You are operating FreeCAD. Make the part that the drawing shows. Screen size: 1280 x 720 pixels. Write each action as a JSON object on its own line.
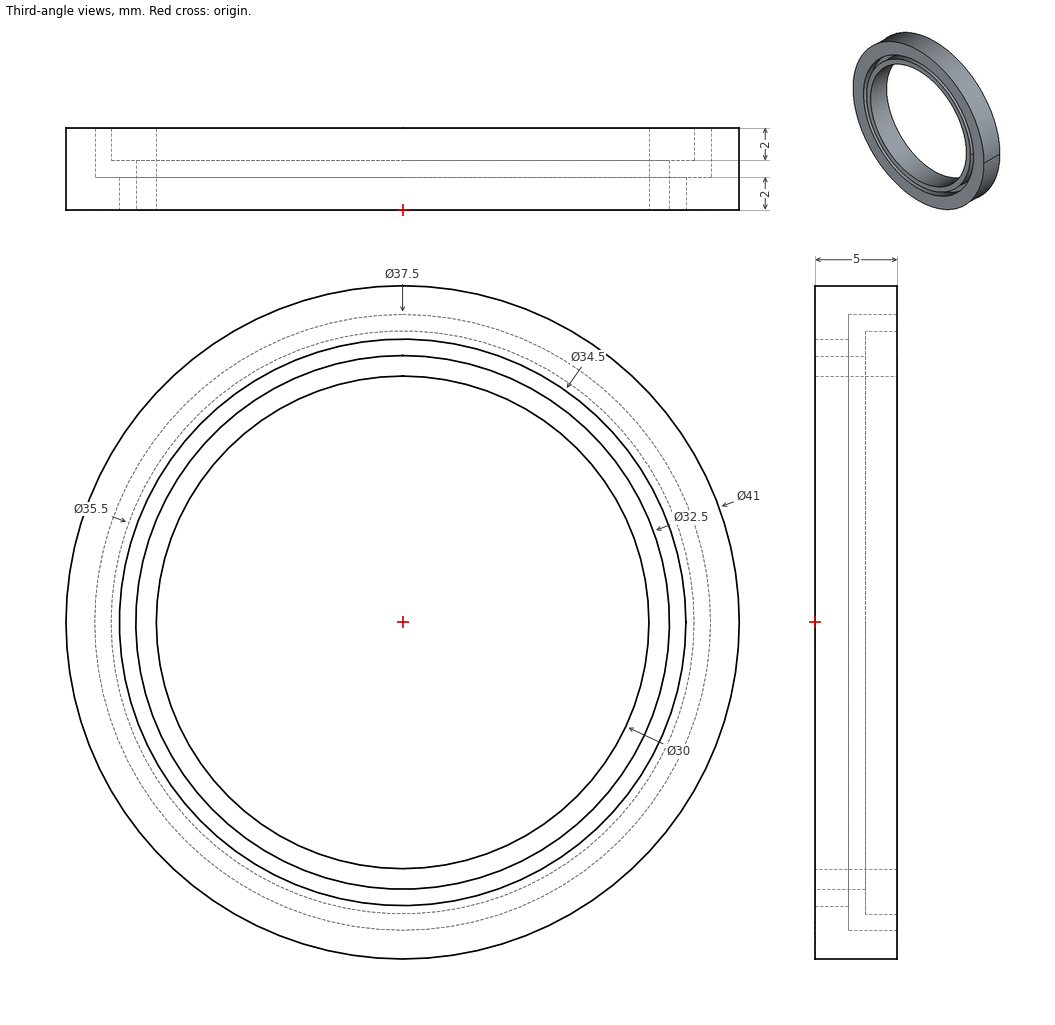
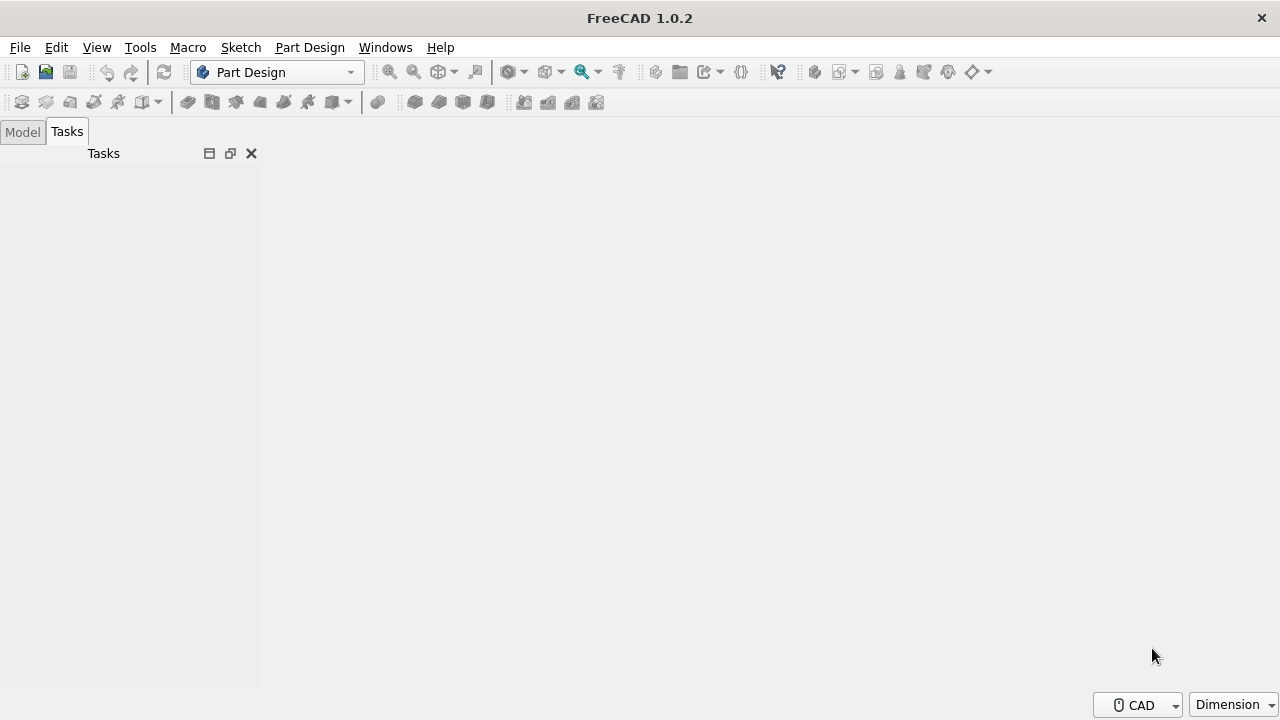
{"action": "key", "text": "ctrl+n"}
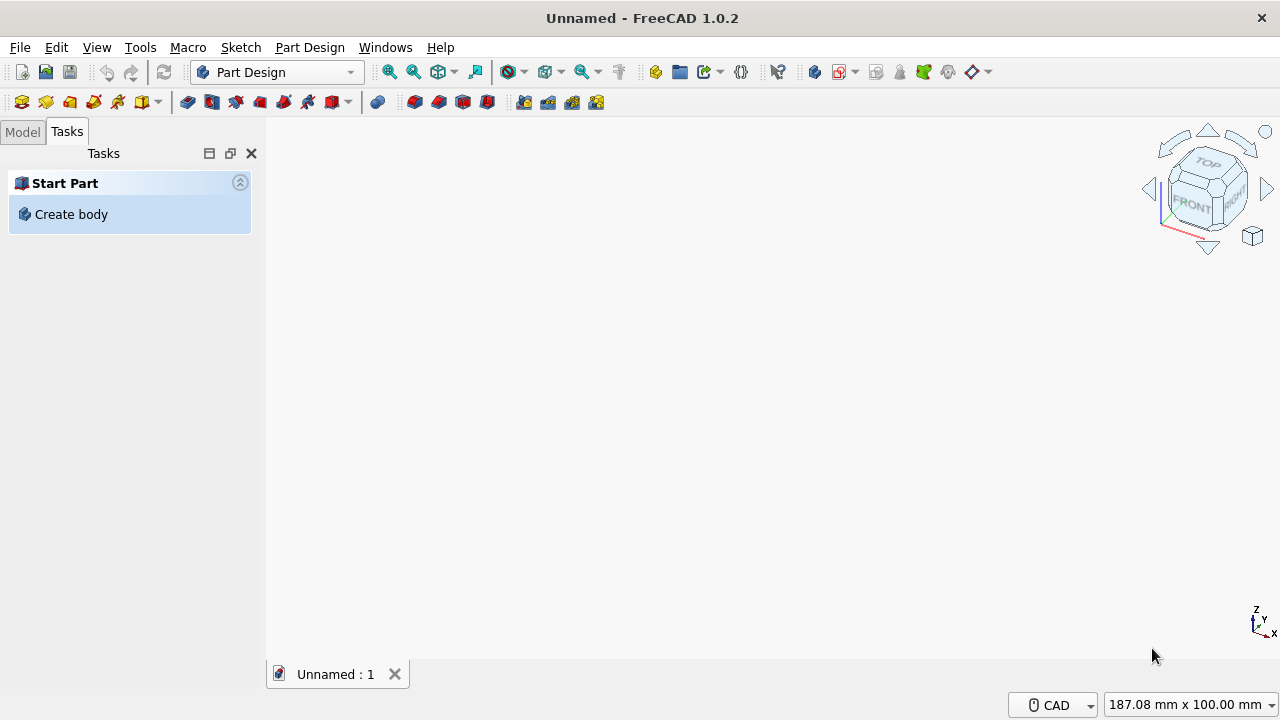
{"action": "left_click", "coordinate": [840, 72]}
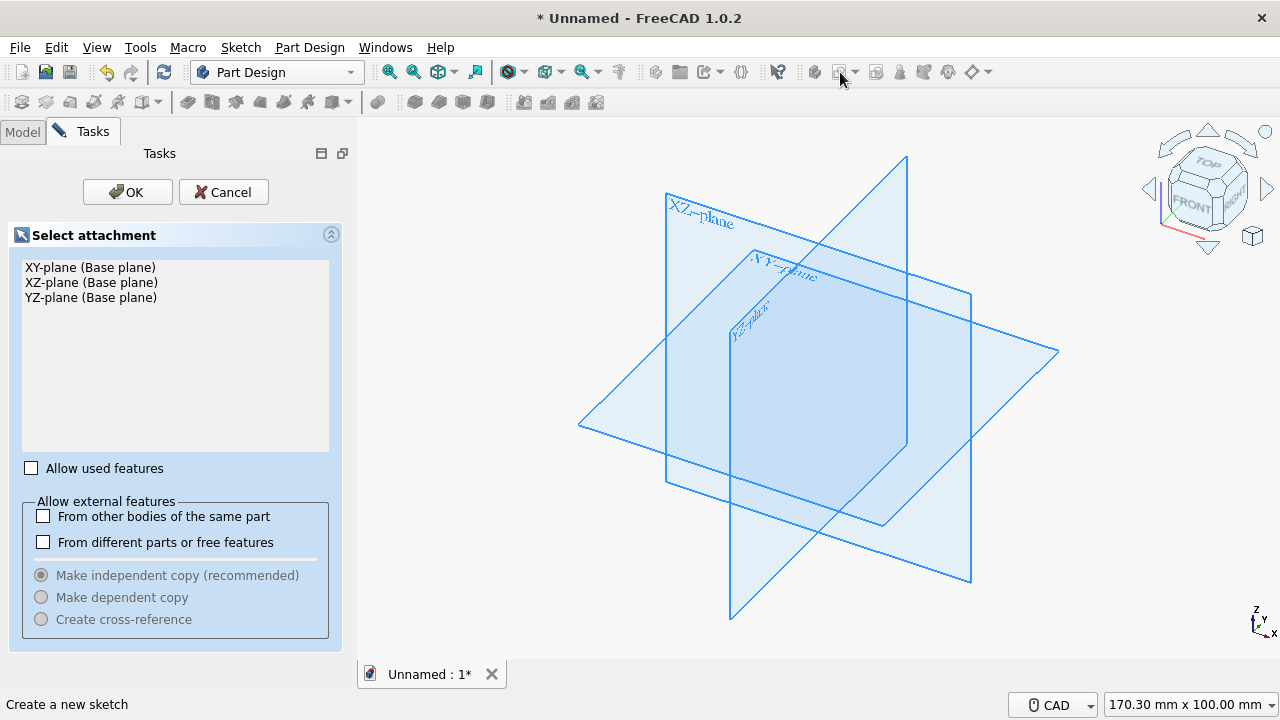
{"action": "left_click", "coordinate": [82, 282]}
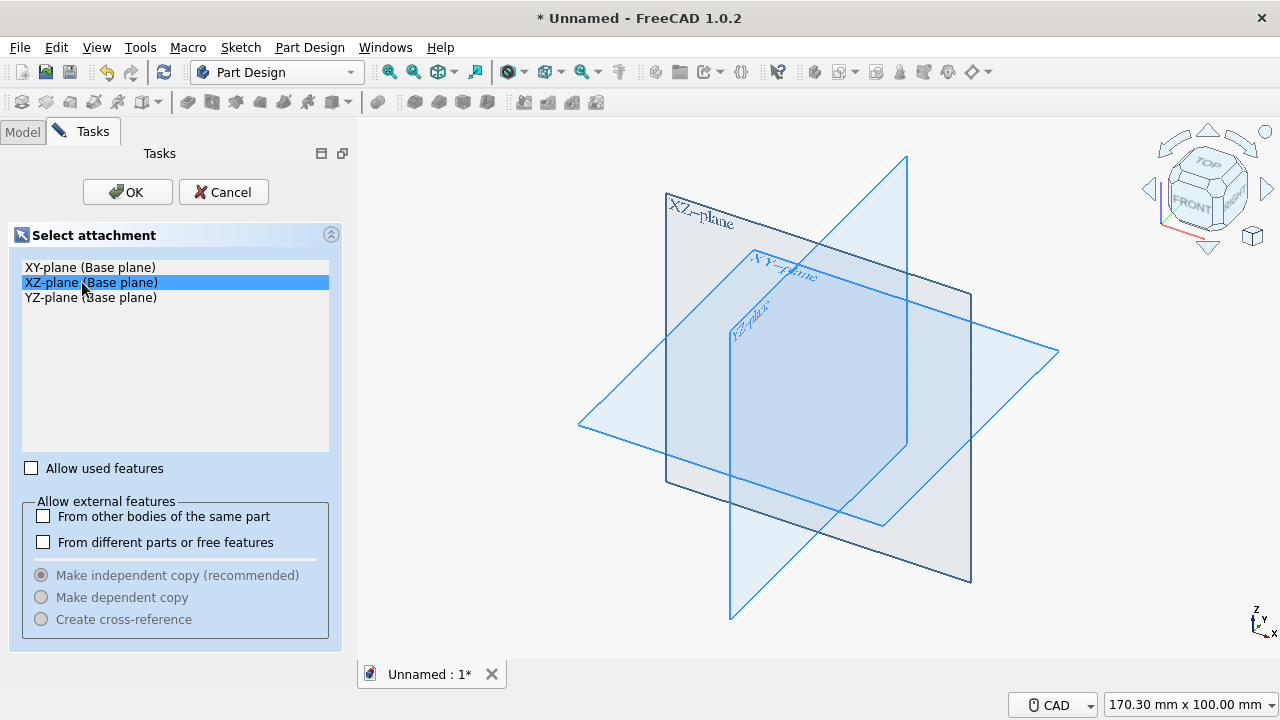
{"action": "left_click", "coordinate": [128, 192]}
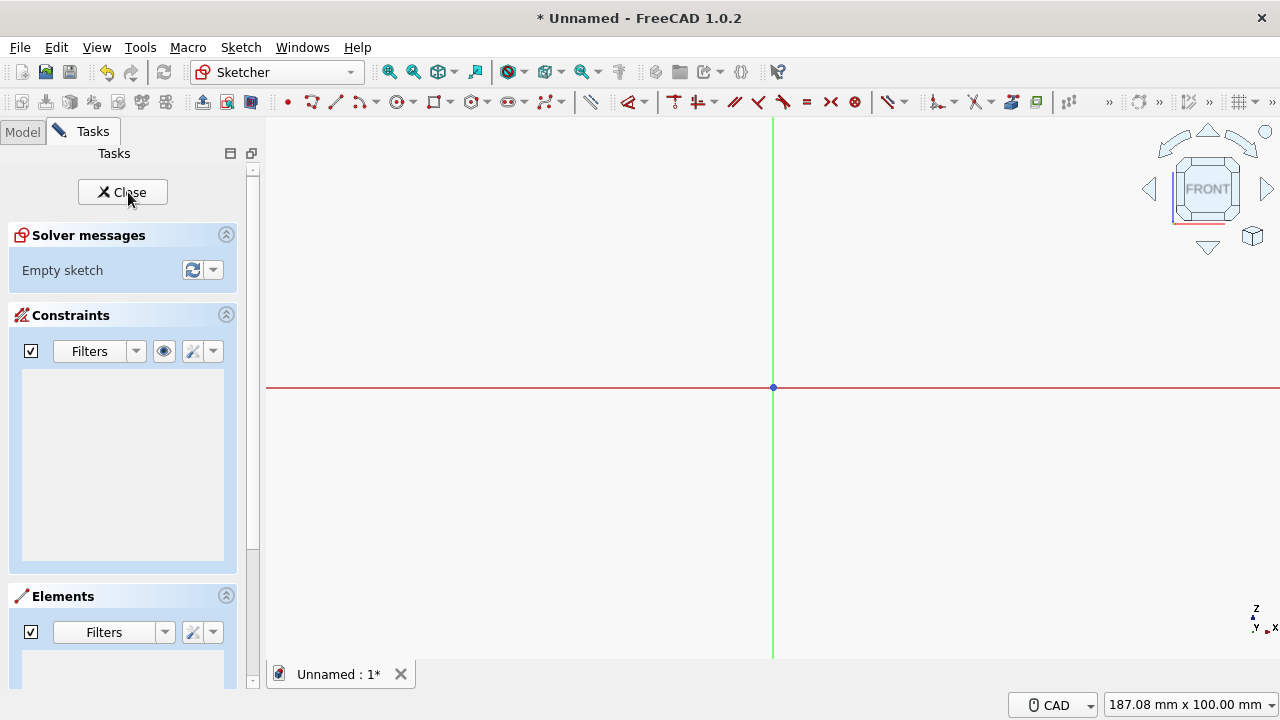
{"action": "scroll", "coordinate": [856, 388], "scroll_direction": "up", "scroll_amount": 3}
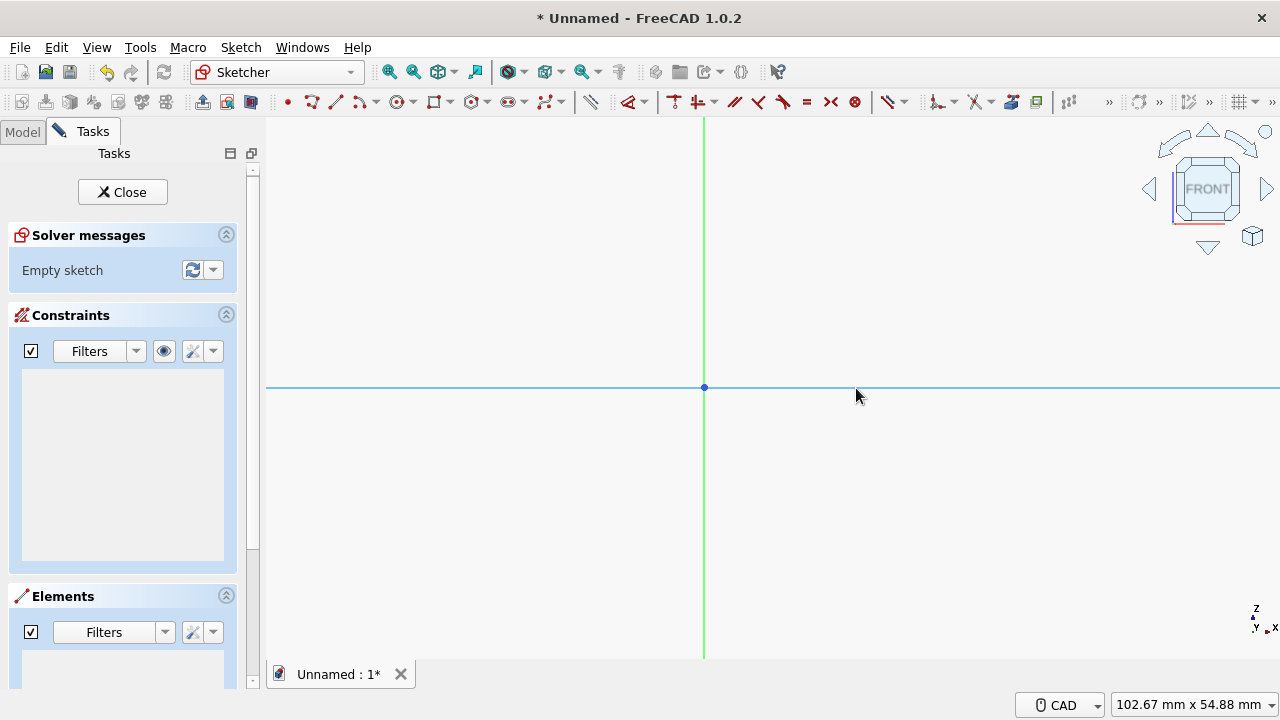
{"action": "key", "text": "g c"}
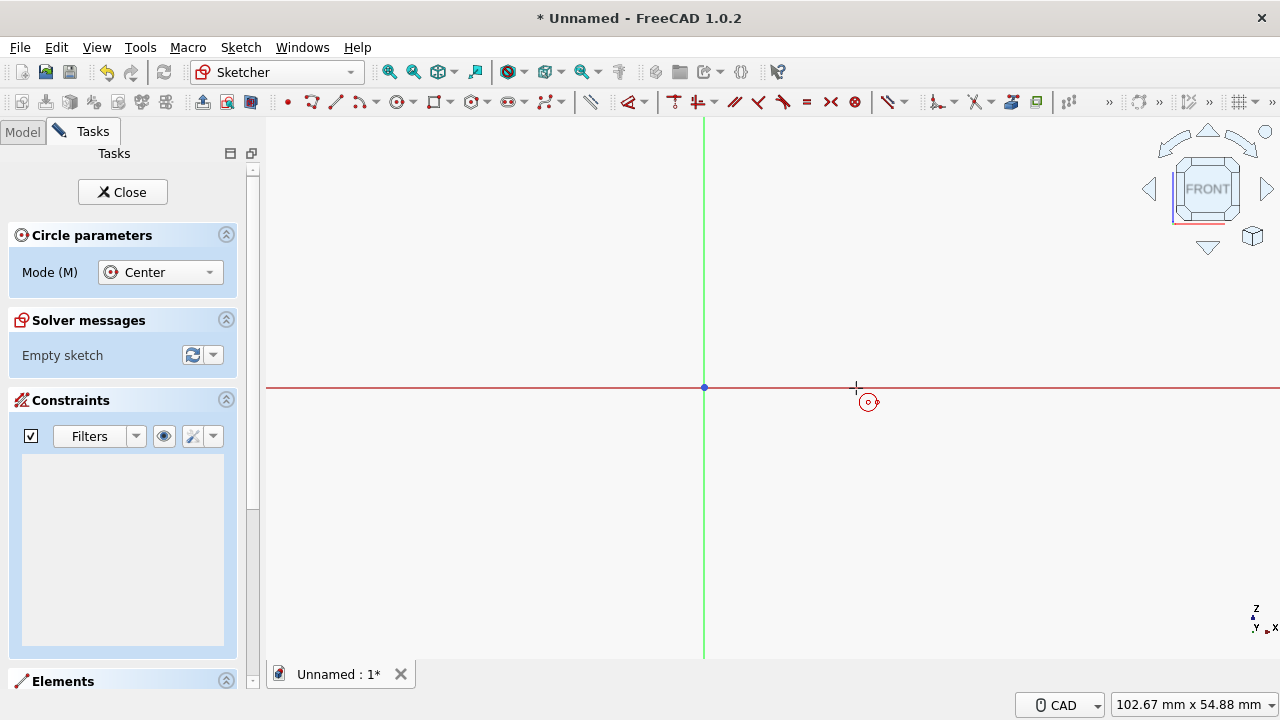
{"action": "left_click", "coordinate": [704, 388]}
{"action": "mouse_move", "coordinate": [818, 274]}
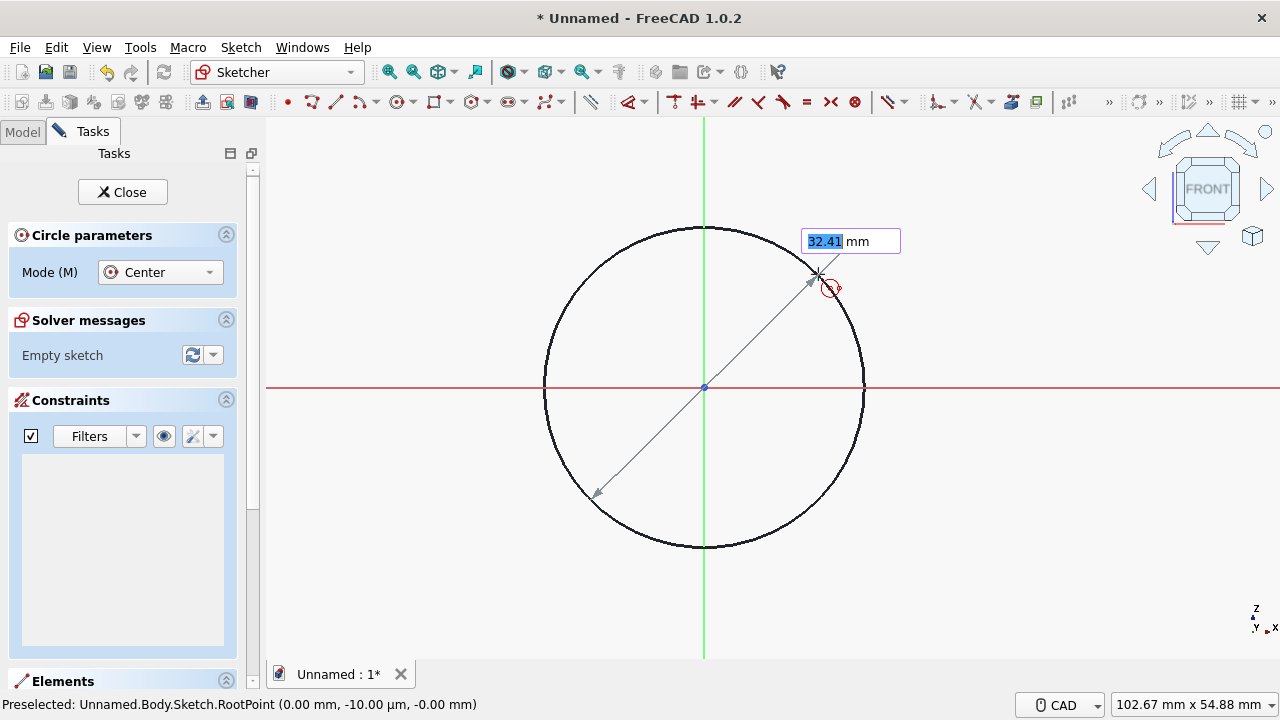
{"action": "type", "text": "32.5"}
{"action": "key", "text": "Return"}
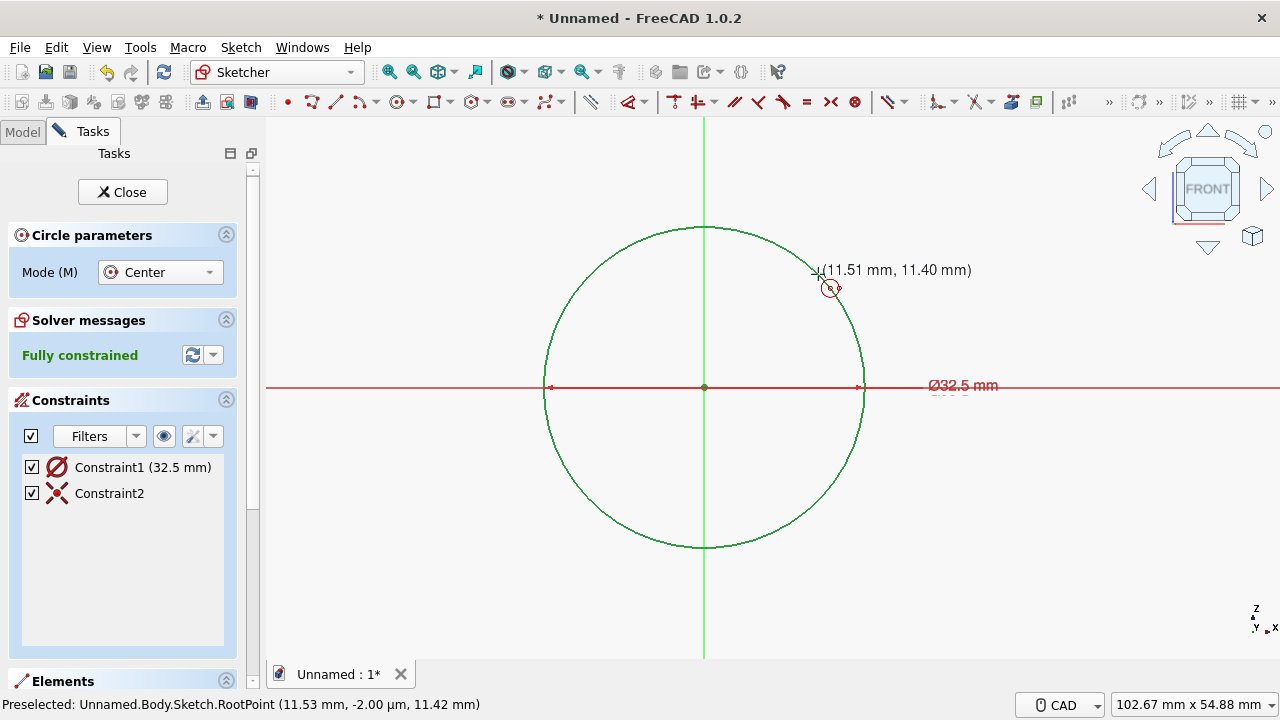
{"action": "left_click", "coordinate": [704, 388]}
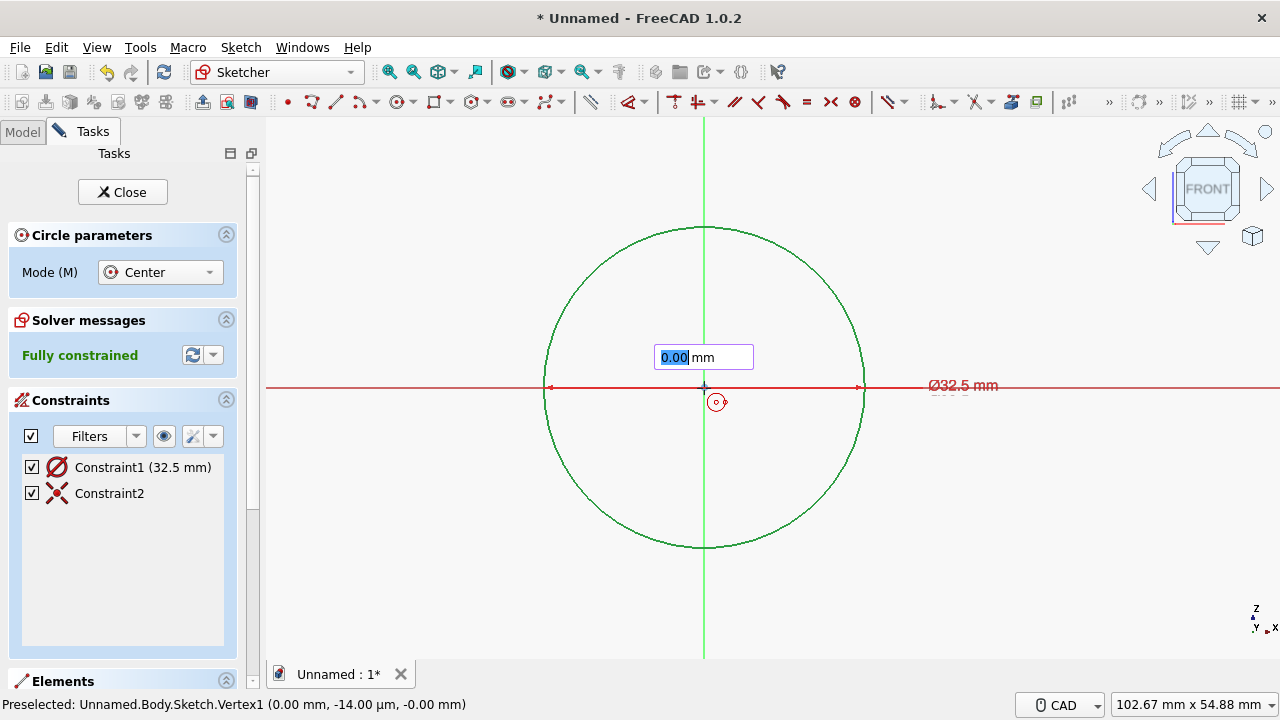
{"action": "scroll", "coordinate": [809, 283], "scroll_direction": "up", "scroll_amount": 2}
{"action": "mouse_move", "coordinate": [809, 283]}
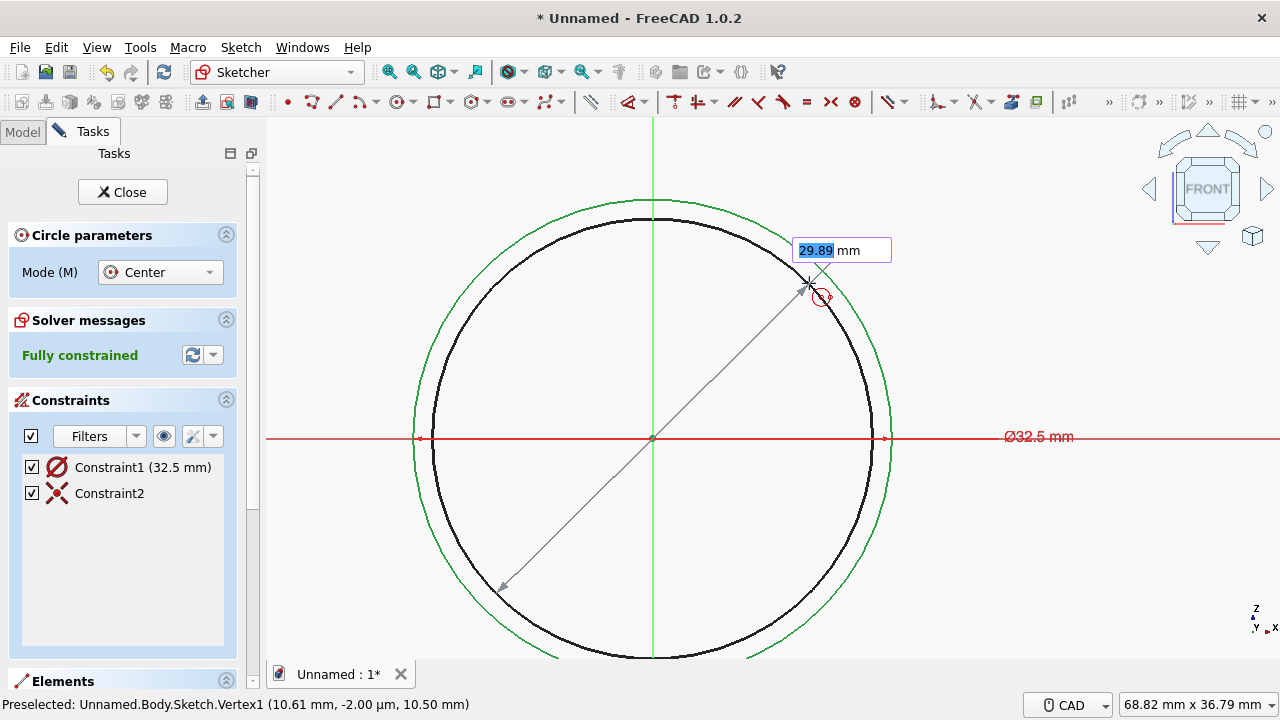
{"action": "type", "text": "30"}
{"action": "key", "text": "Return"}
{"action": "key", "text": "Escape"}